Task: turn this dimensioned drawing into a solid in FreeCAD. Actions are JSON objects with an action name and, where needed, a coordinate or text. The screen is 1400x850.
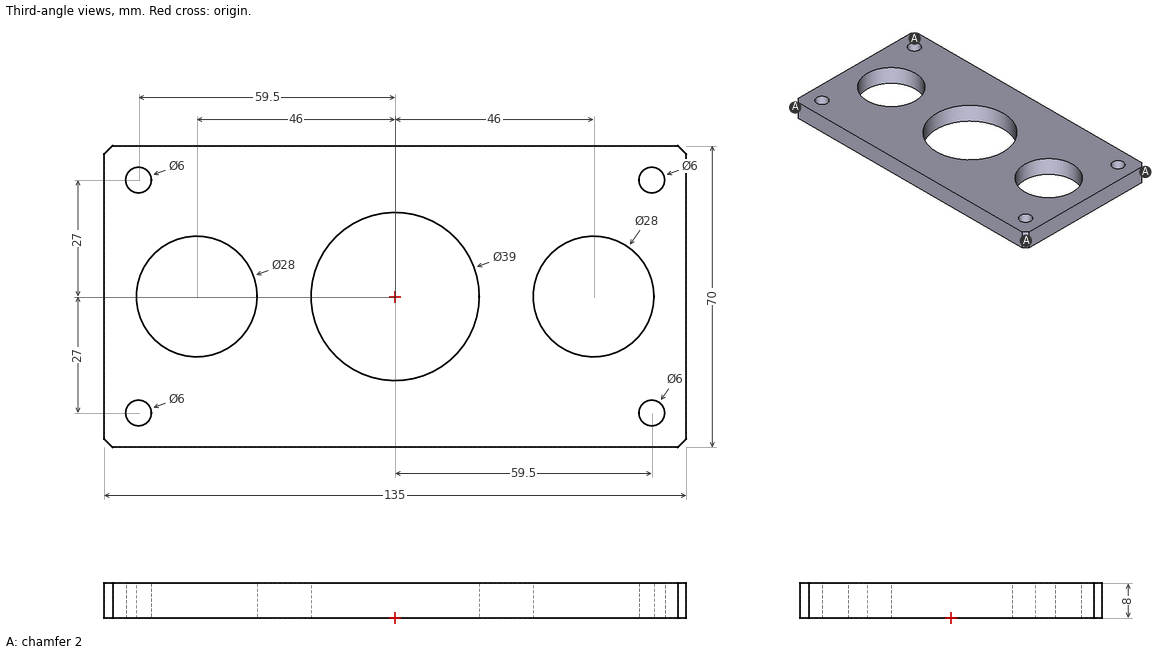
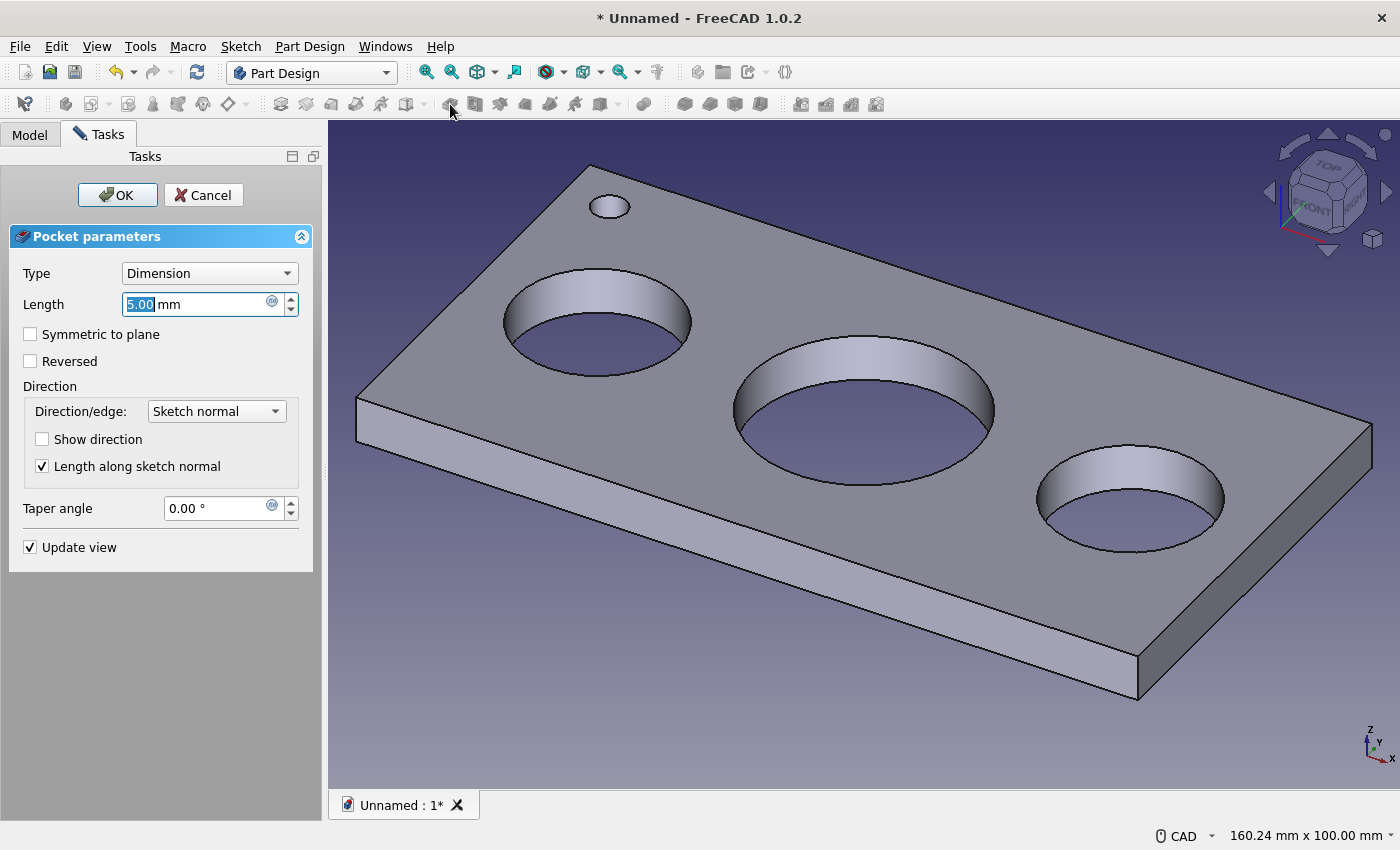
{"action": "left_click", "coordinate": [210, 274]}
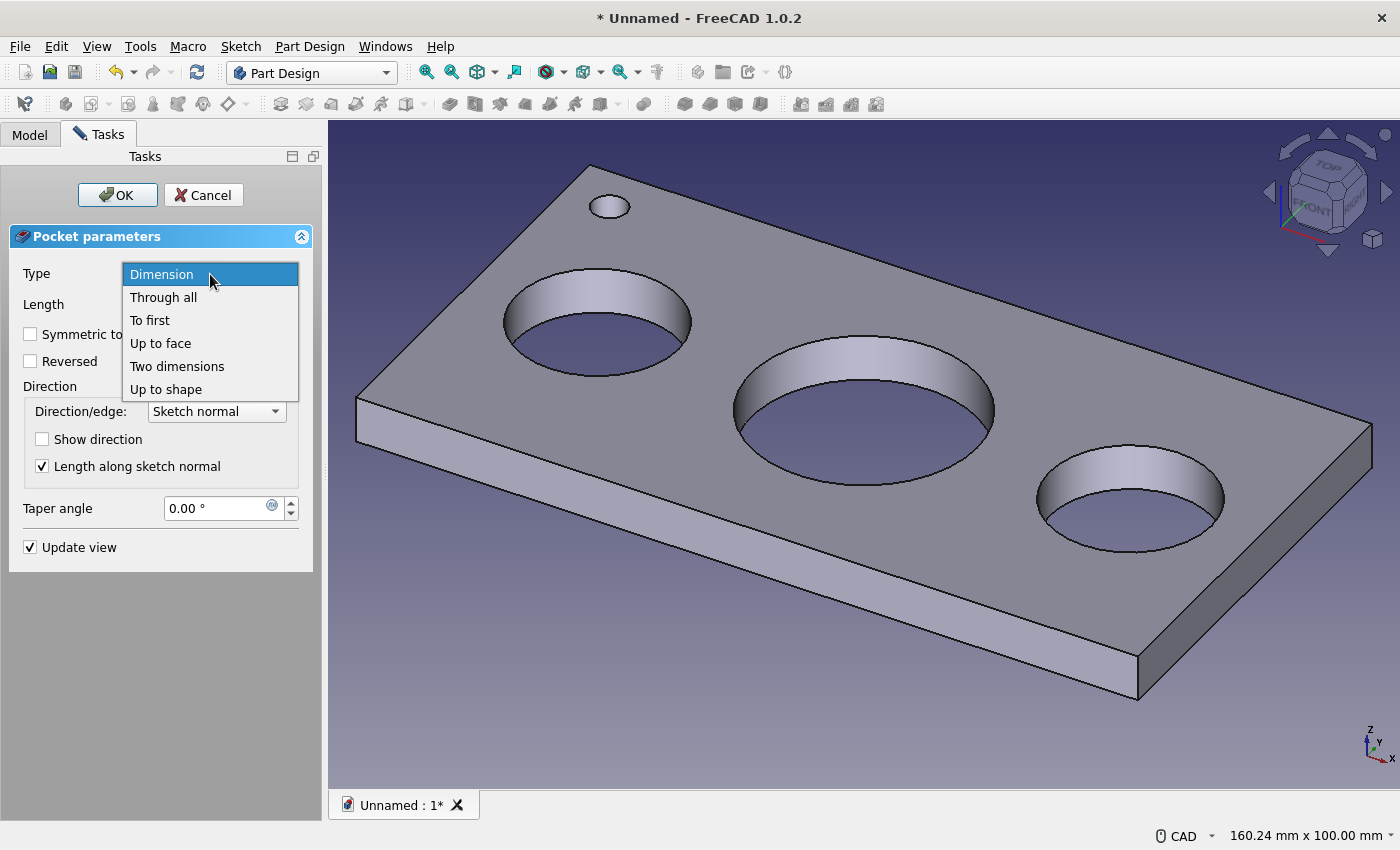
{"action": "left_click", "coordinate": [208, 320]}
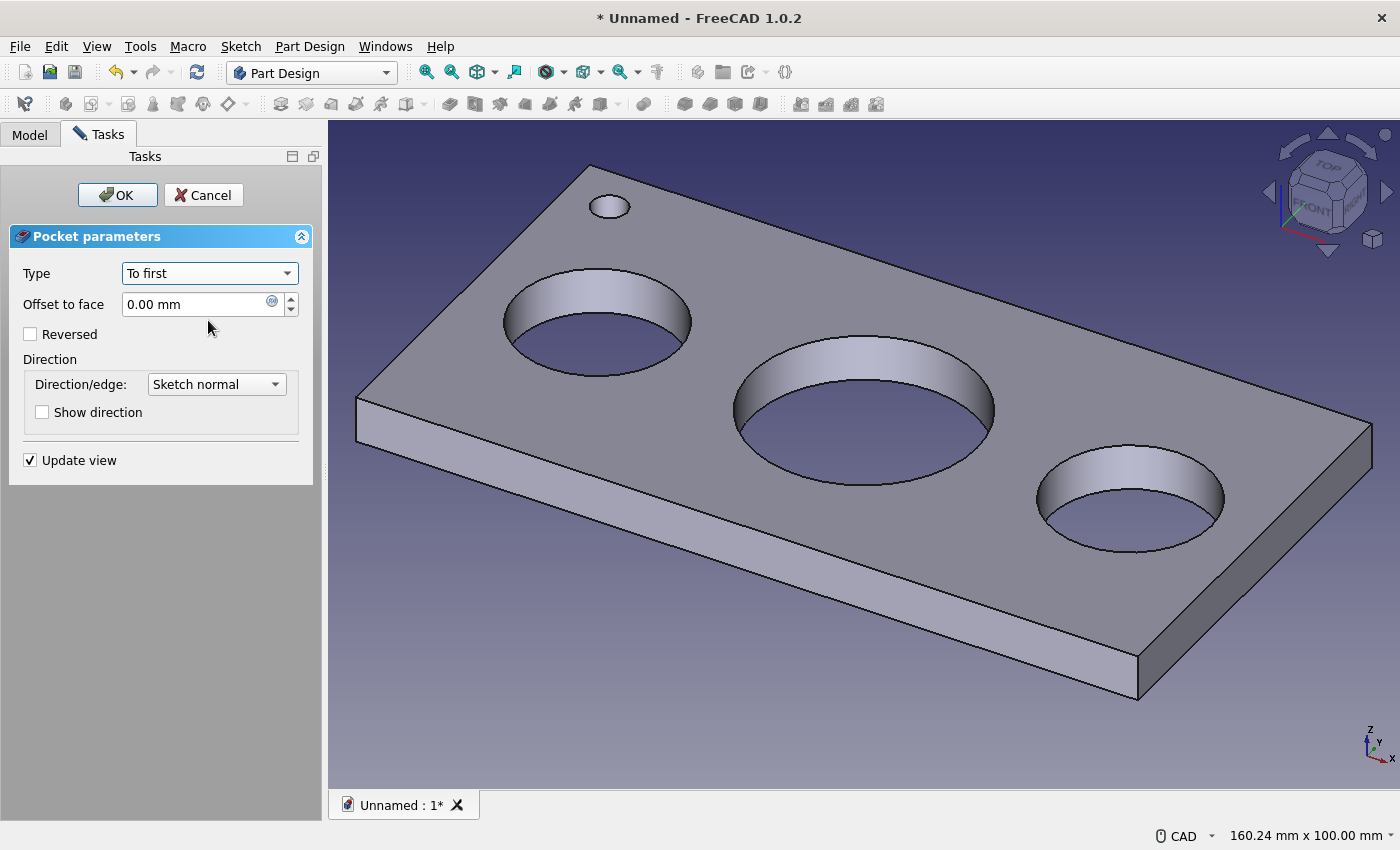
{"action": "left_click", "coordinate": [118, 195]}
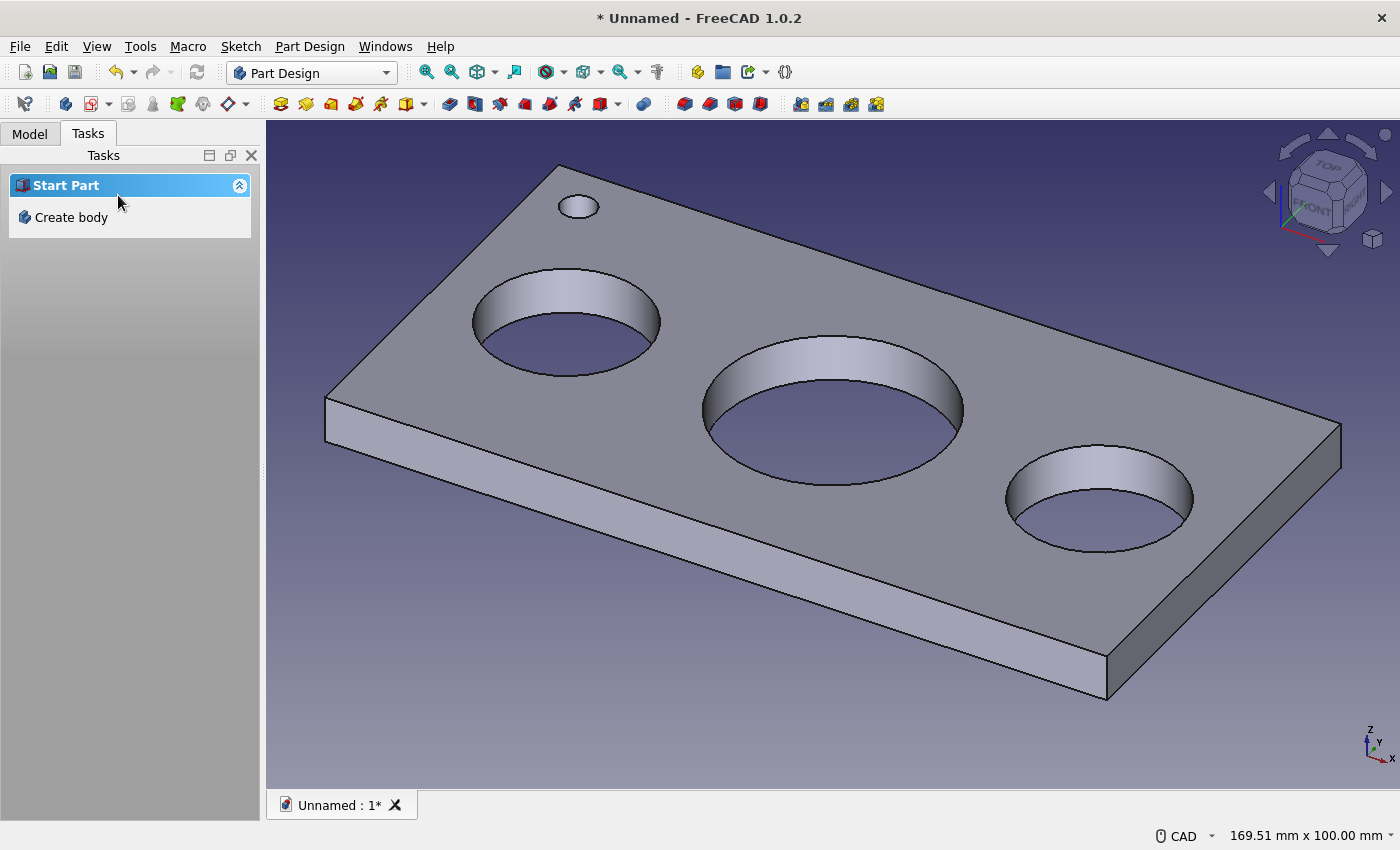
{"action": "left_click", "coordinate": [431, 365]}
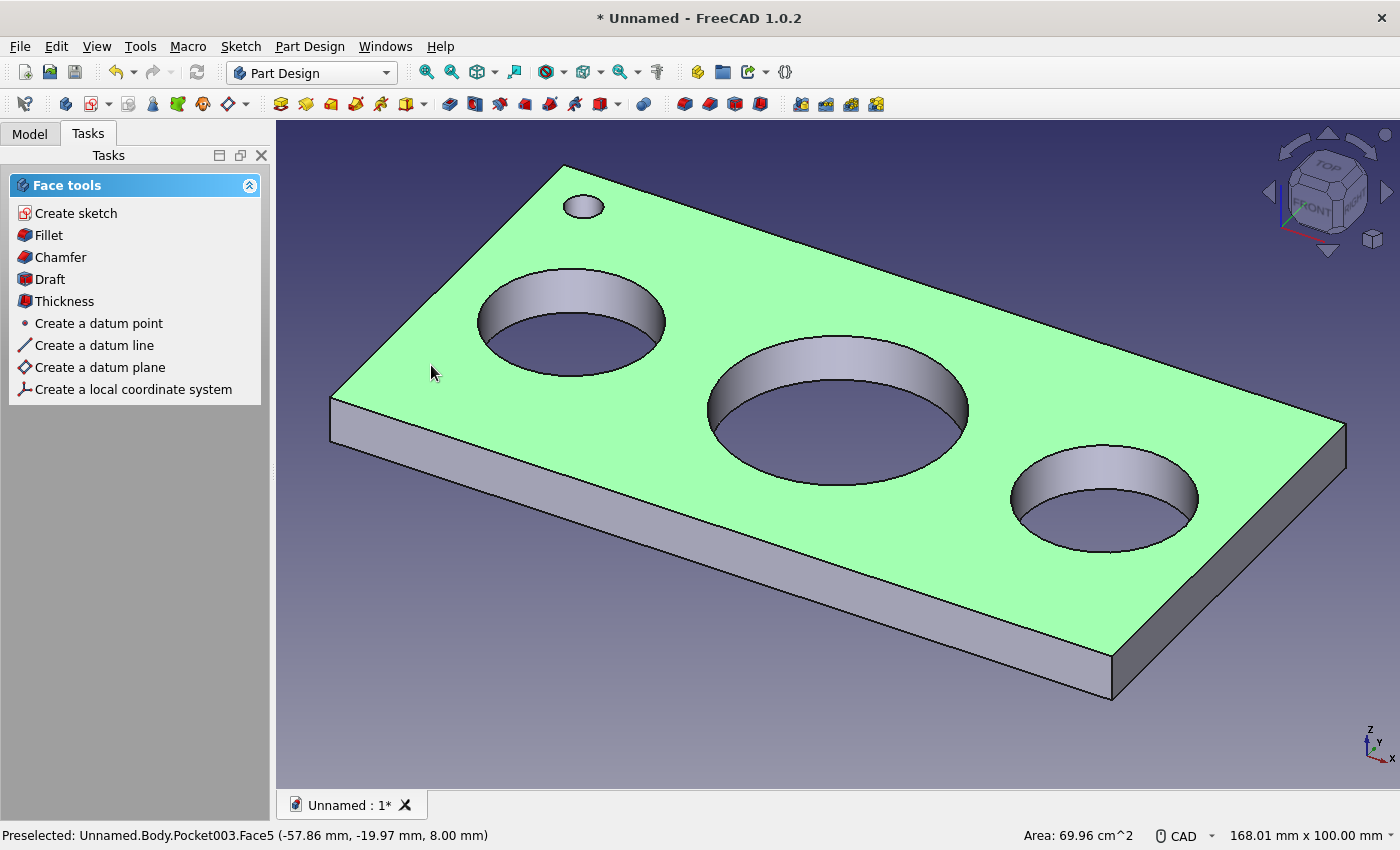
{"action": "left_click", "coordinate": [90, 104]}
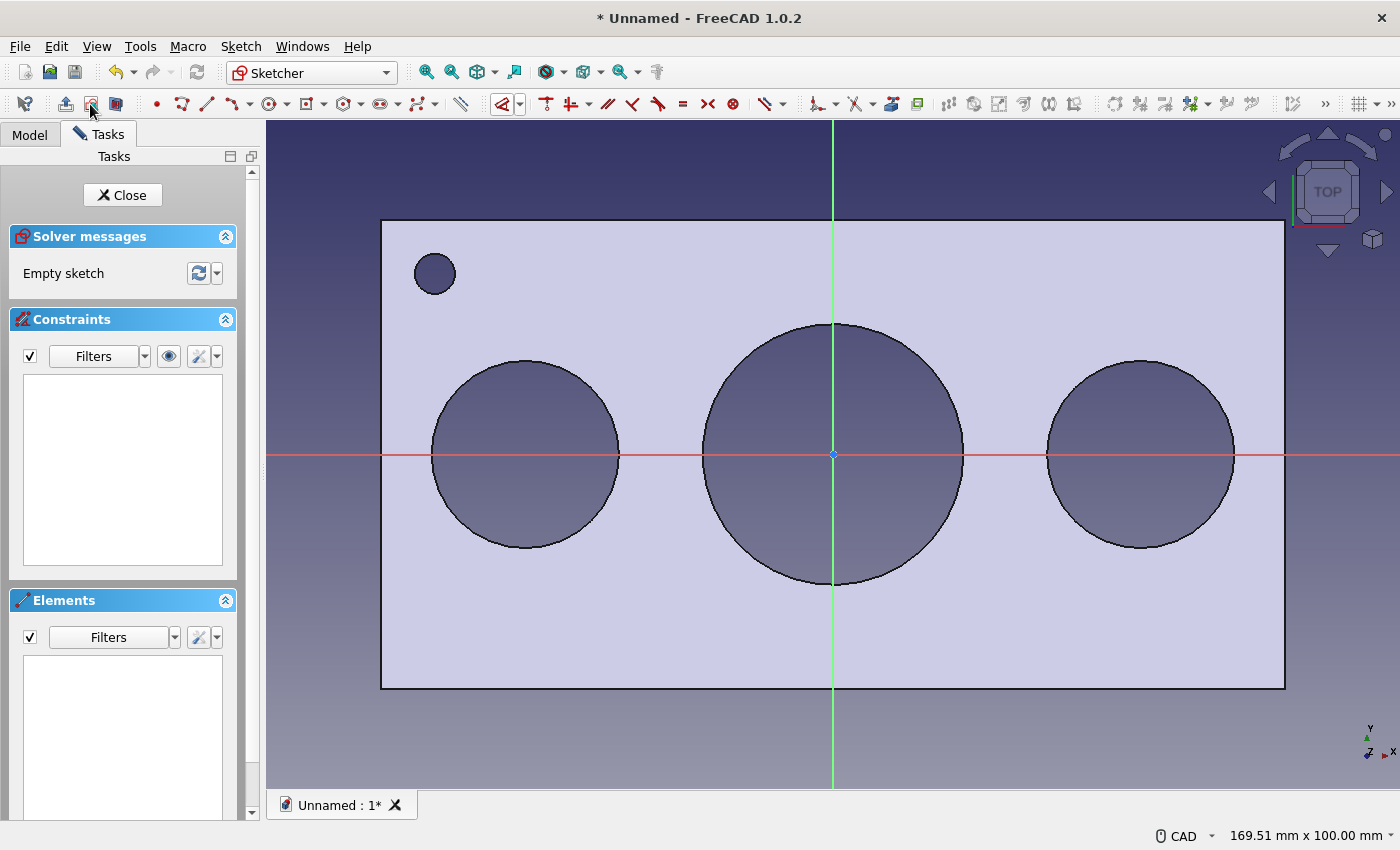
{"action": "scroll", "coordinate": [402, 653], "scroll_direction": "up", "scroll_amount": 12}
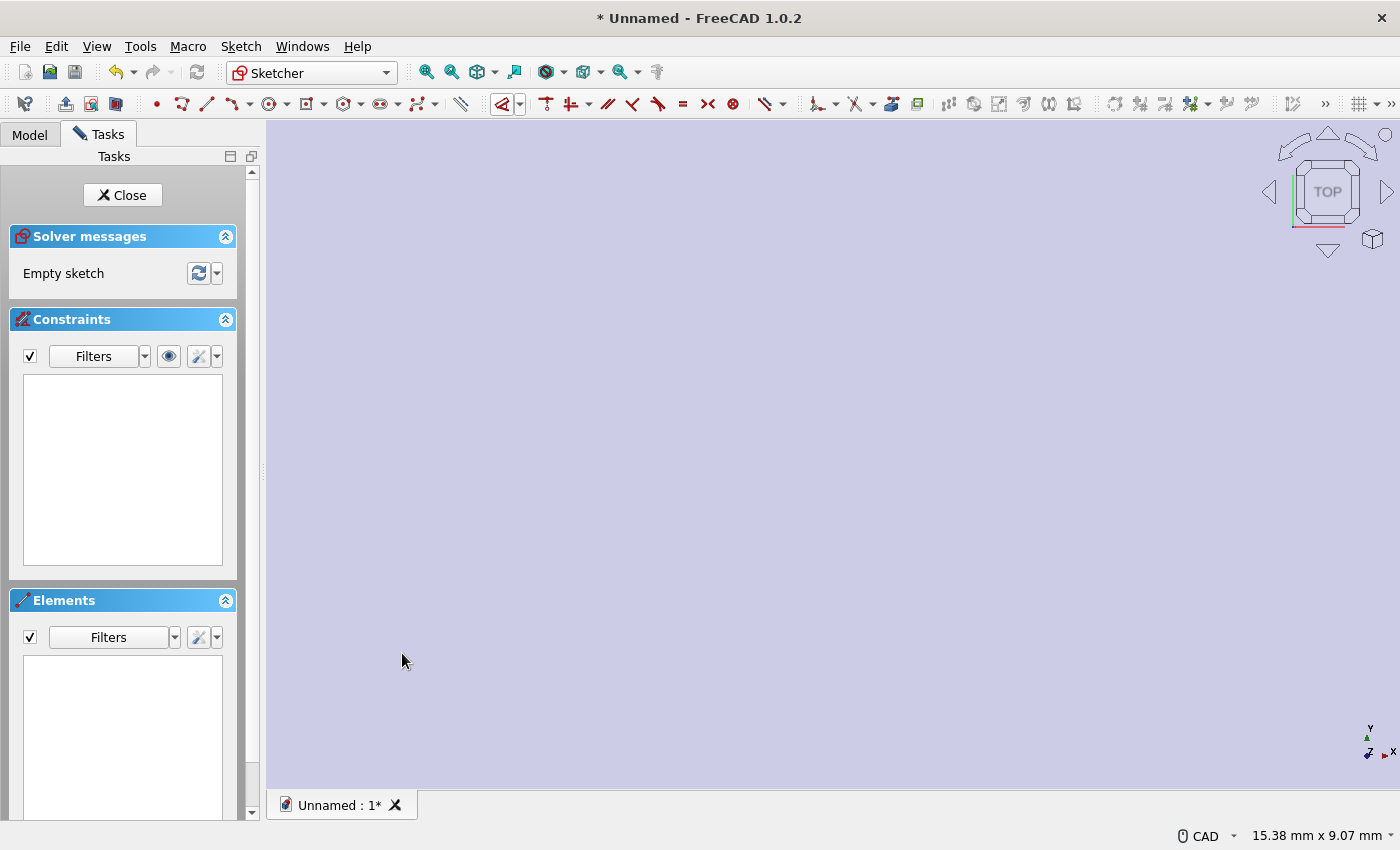
{"action": "key", "text": "g c"}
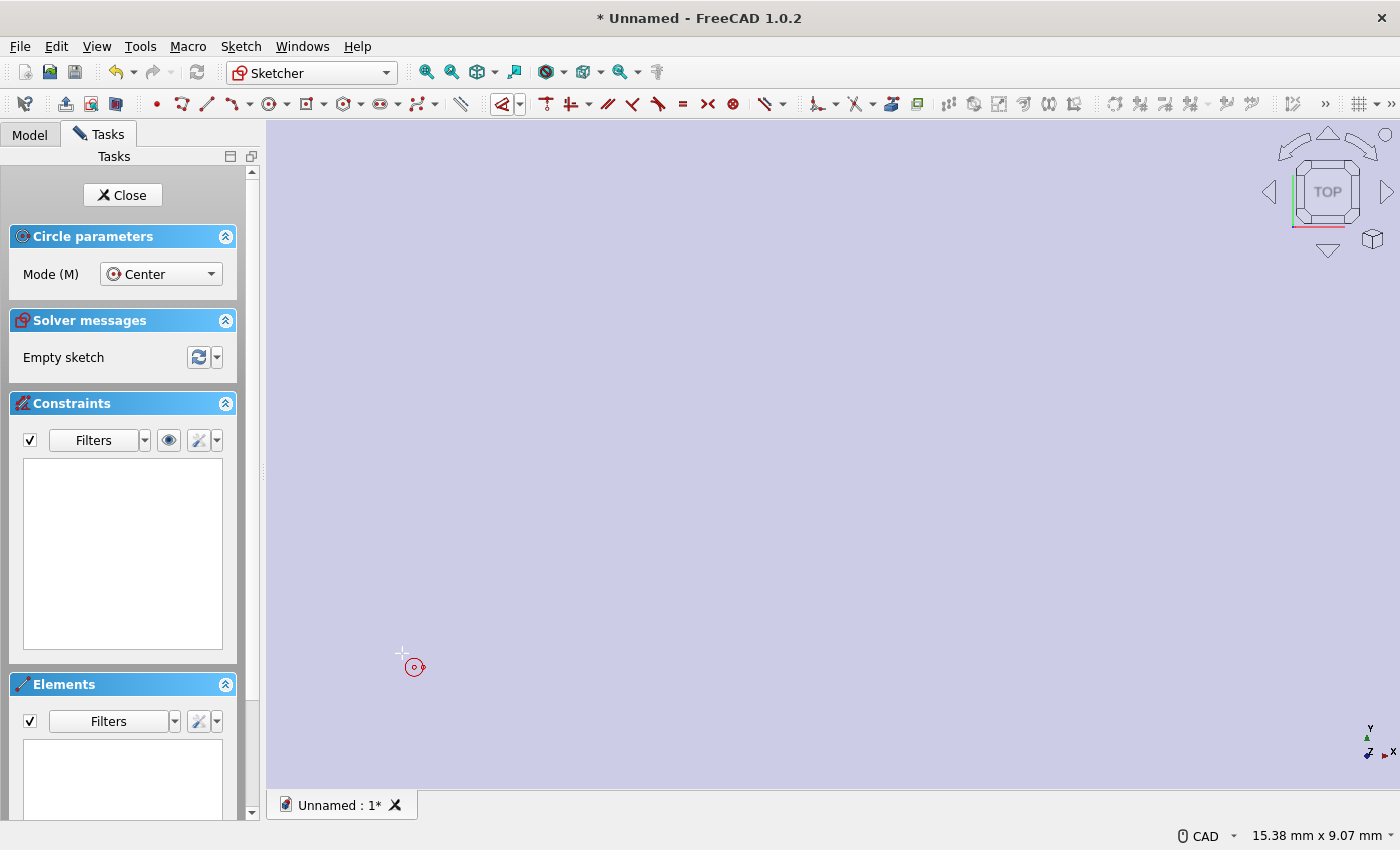
{"action": "left_click", "coordinate": [764, 448]}
{"action": "left_click", "coordinate": [920, 292]}
{"action": "key", "text": "Escape"}